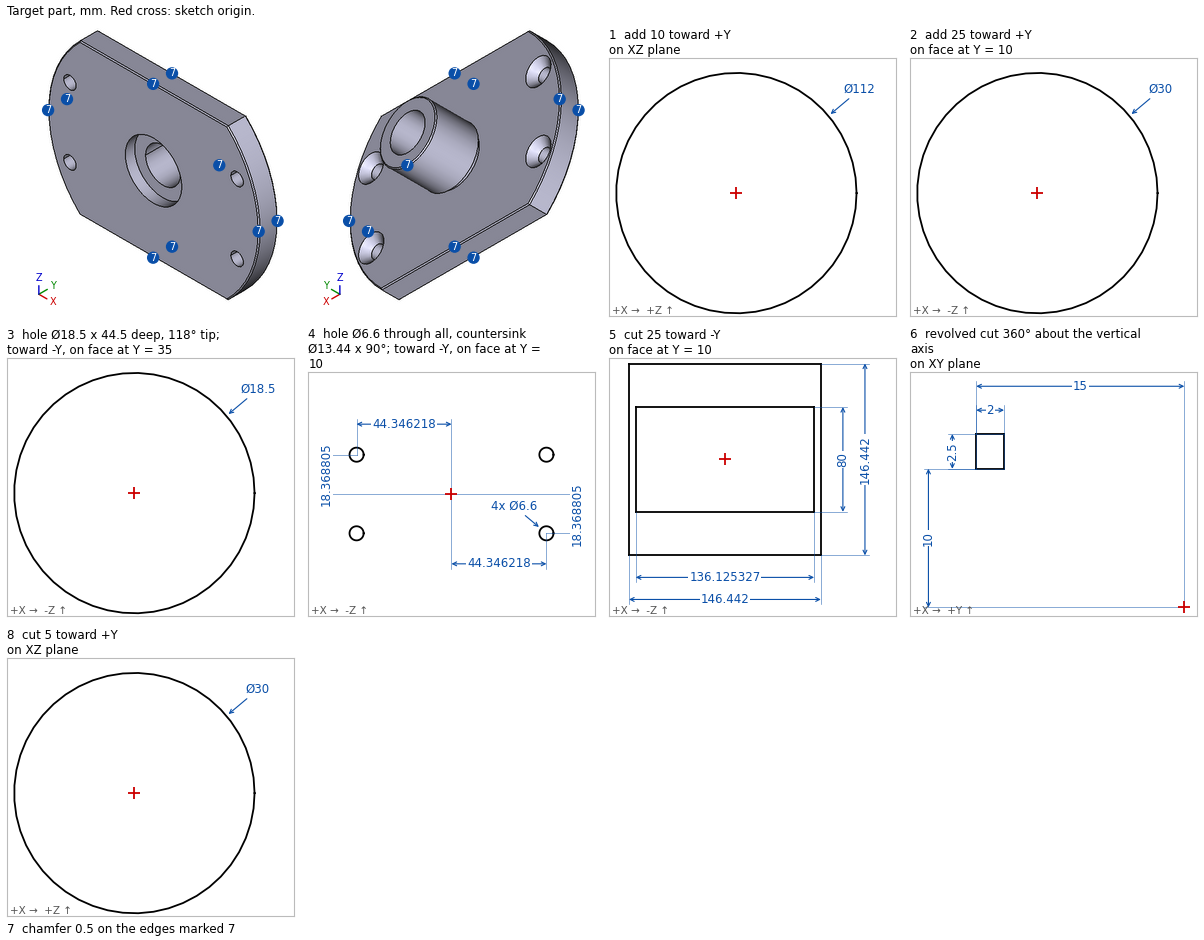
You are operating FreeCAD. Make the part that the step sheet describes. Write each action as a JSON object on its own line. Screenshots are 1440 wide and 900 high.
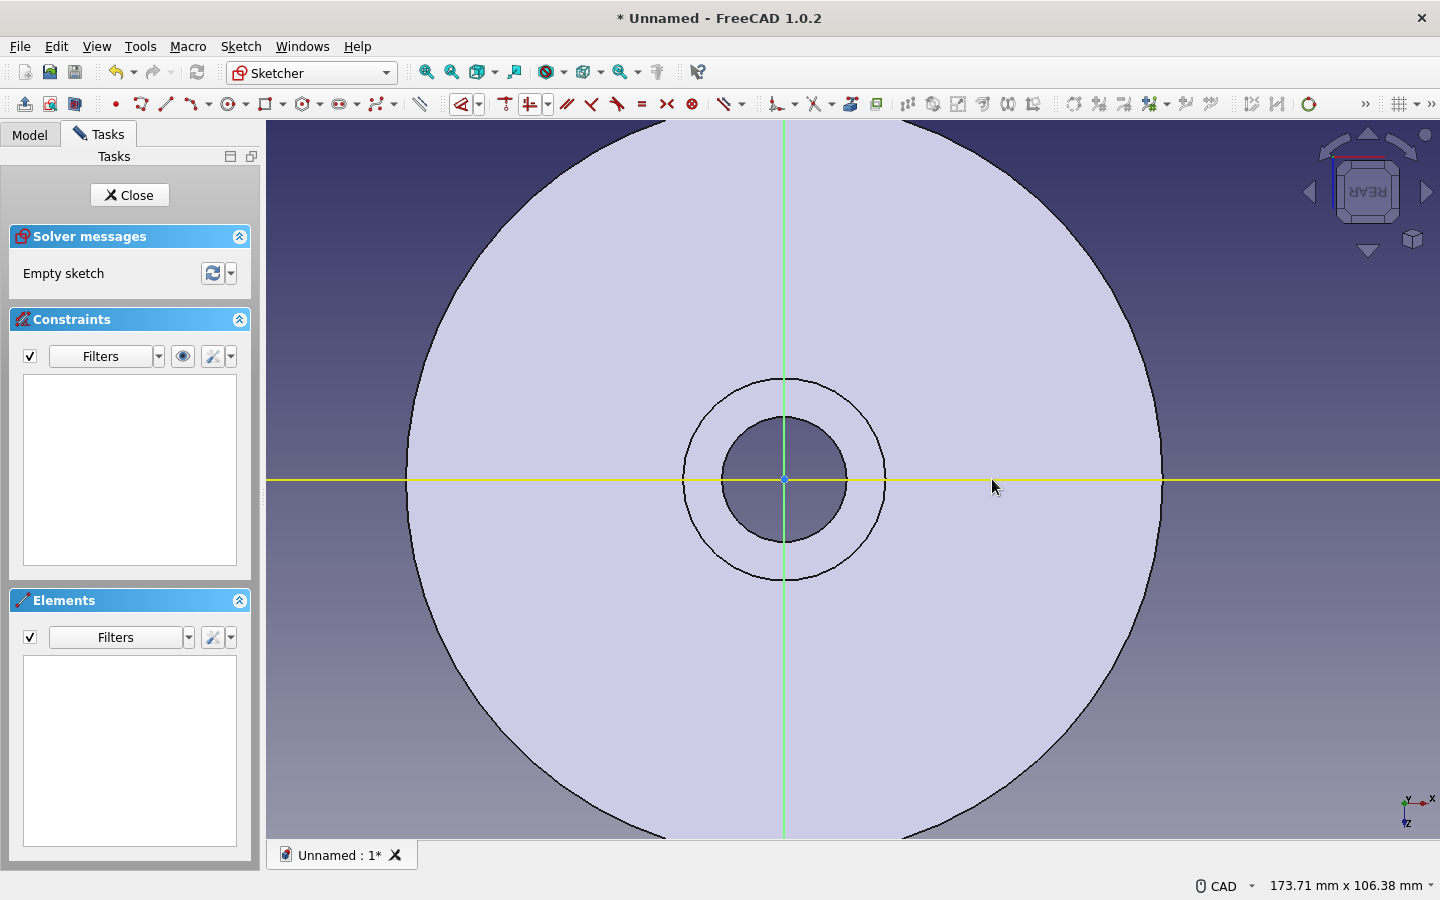
{"action": "left_click", "coordinate": [228, 104]}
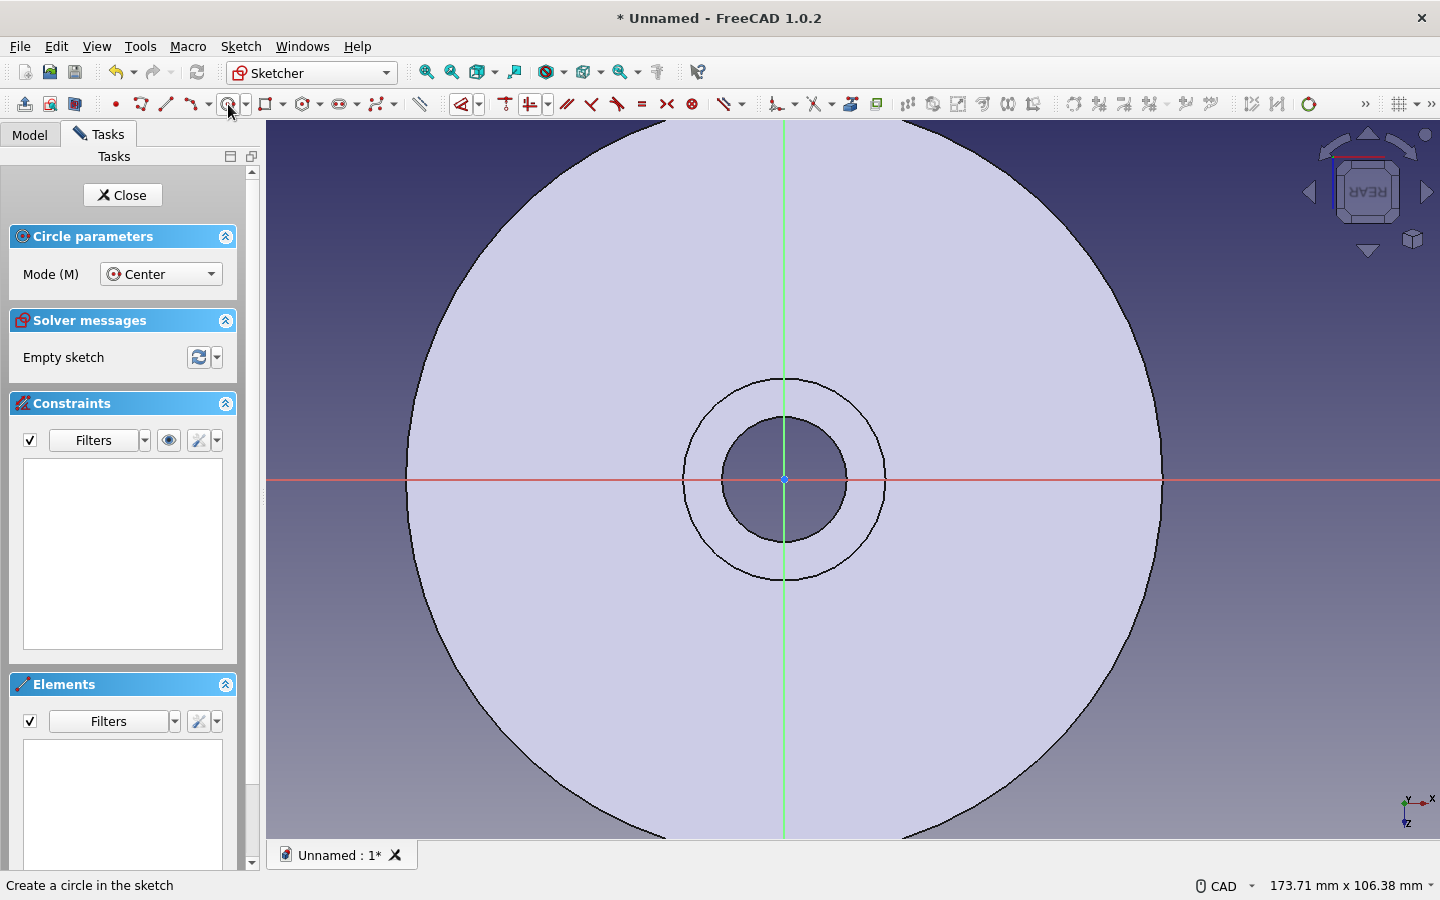
{"action": "left_click", "coordinate": [1084, 604]}
{"action": "mouse_move", "coordinate": [1100, 588]}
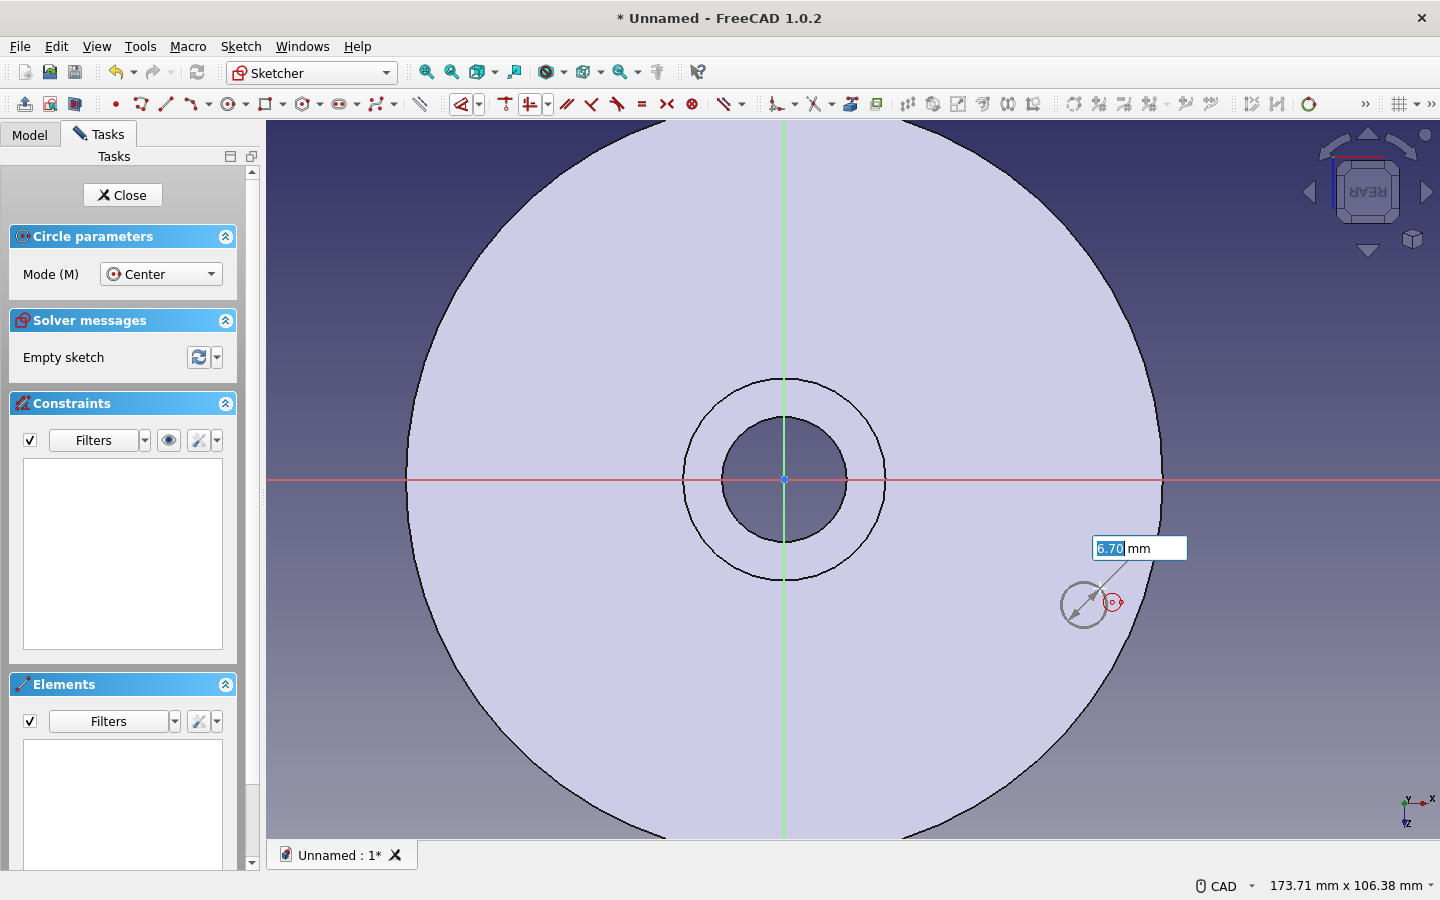
{"action": "type", "text": "6.6"}
{"action": "key", "text": "Return"}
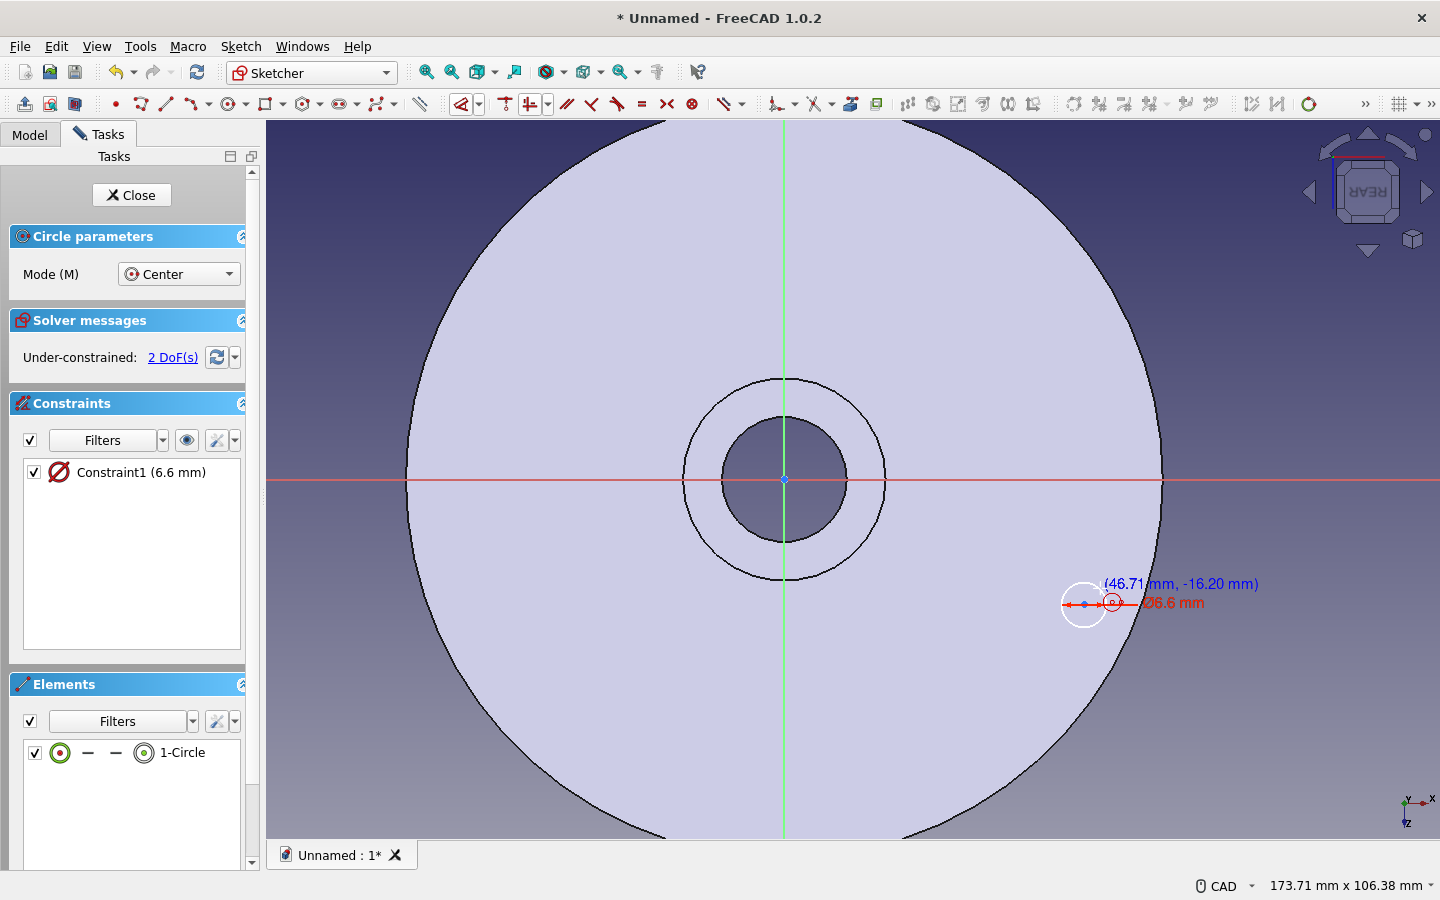
{"action": "left_click", "coordinate": [485, 355]}
{"action": "mouse_move", "coordinate": [500, 340]}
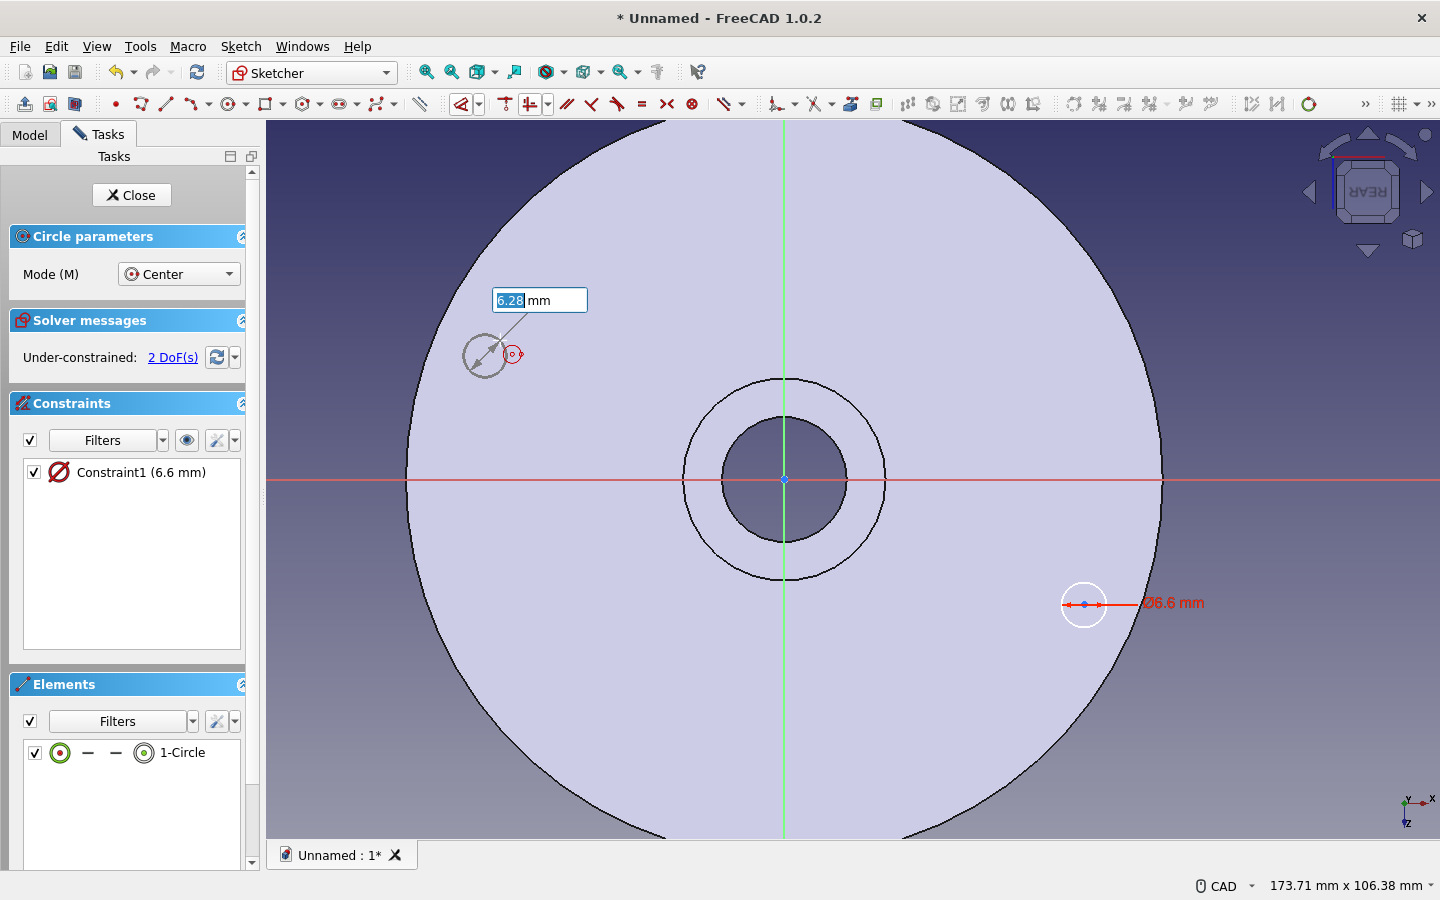
{"action": "type", "text": "6.6"}
{"action": "key", "text": "Return"}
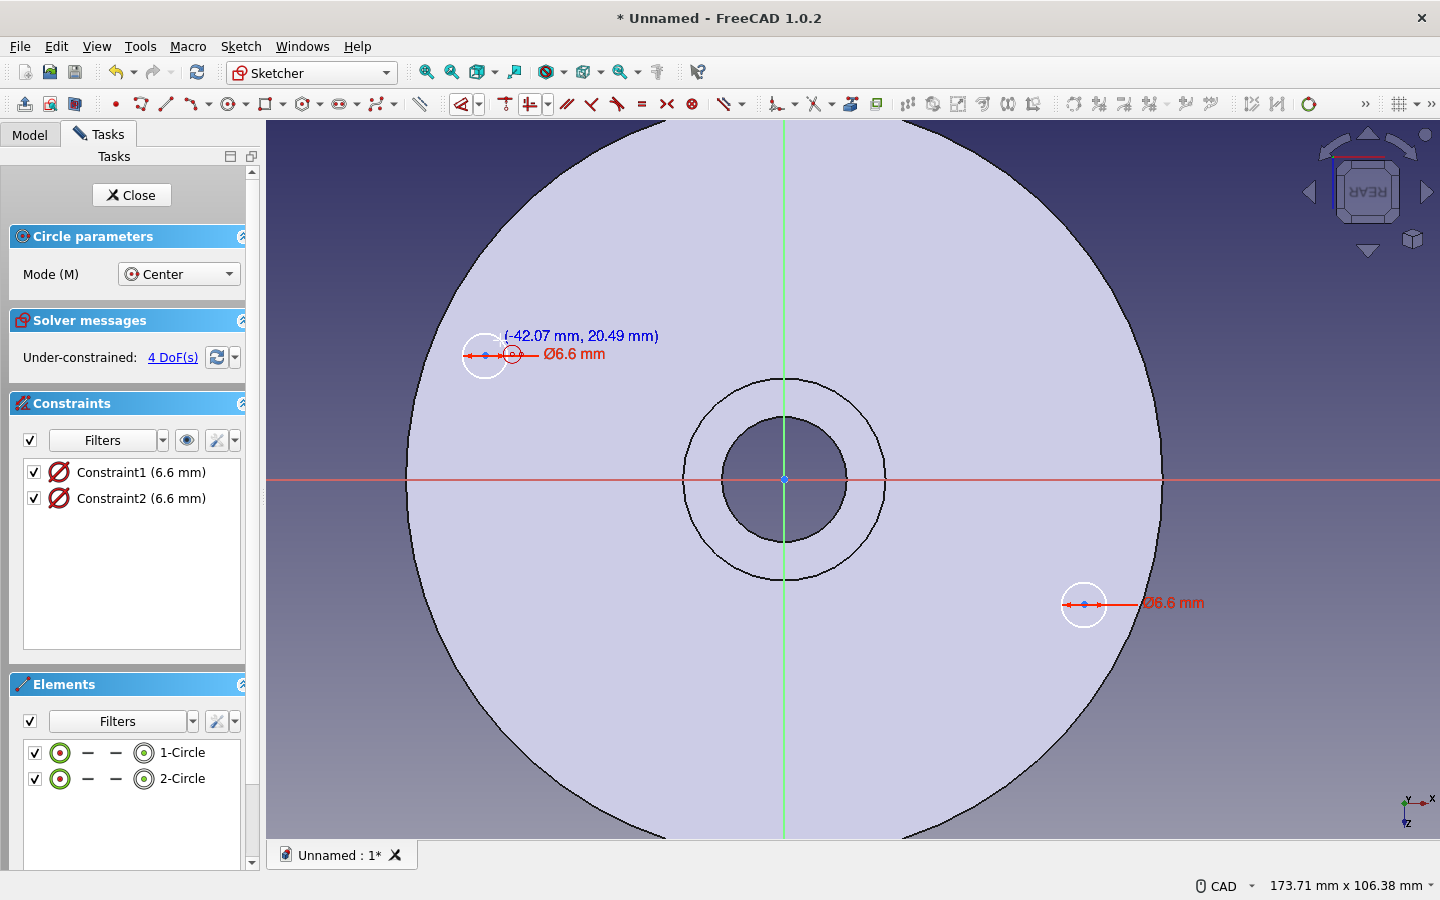
{"action": "left_click", "coordinate": [485, 604]}
{"action": "mouse_move", "coordinate": [500, 588]}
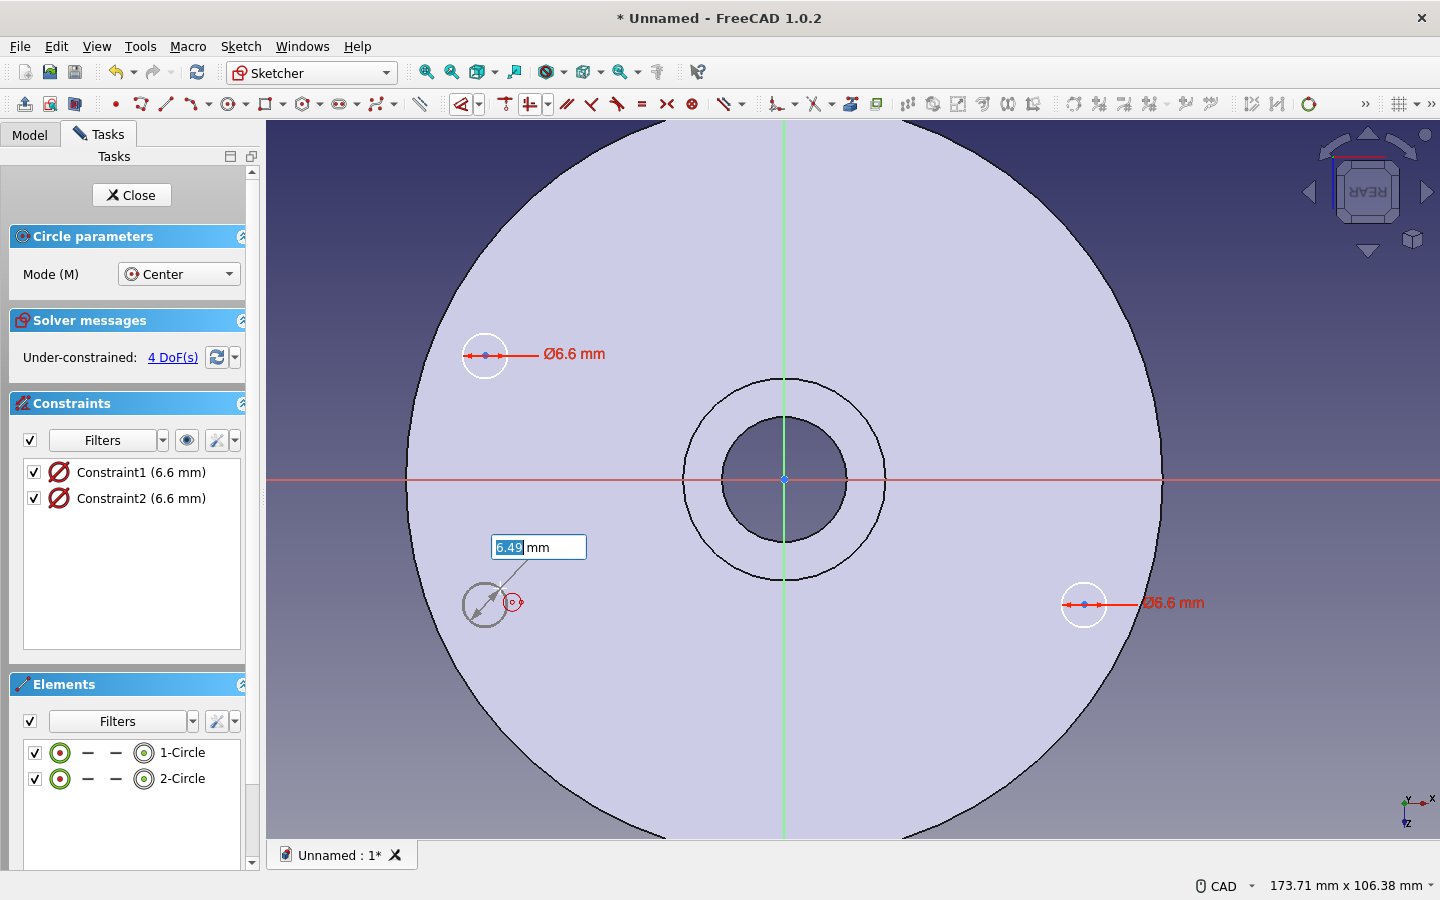
{"action": "type", "text": "6.6"}
{"action": "key", "text": "Return"}